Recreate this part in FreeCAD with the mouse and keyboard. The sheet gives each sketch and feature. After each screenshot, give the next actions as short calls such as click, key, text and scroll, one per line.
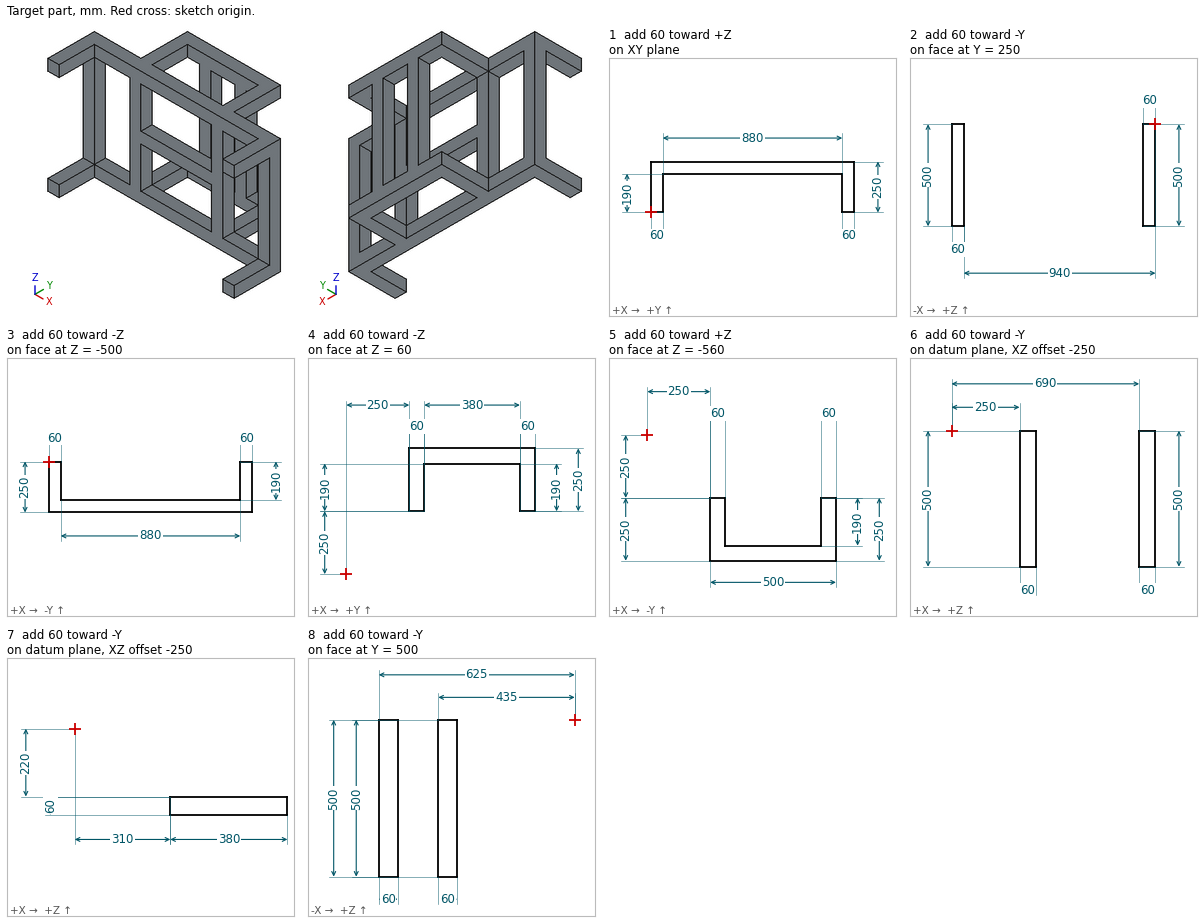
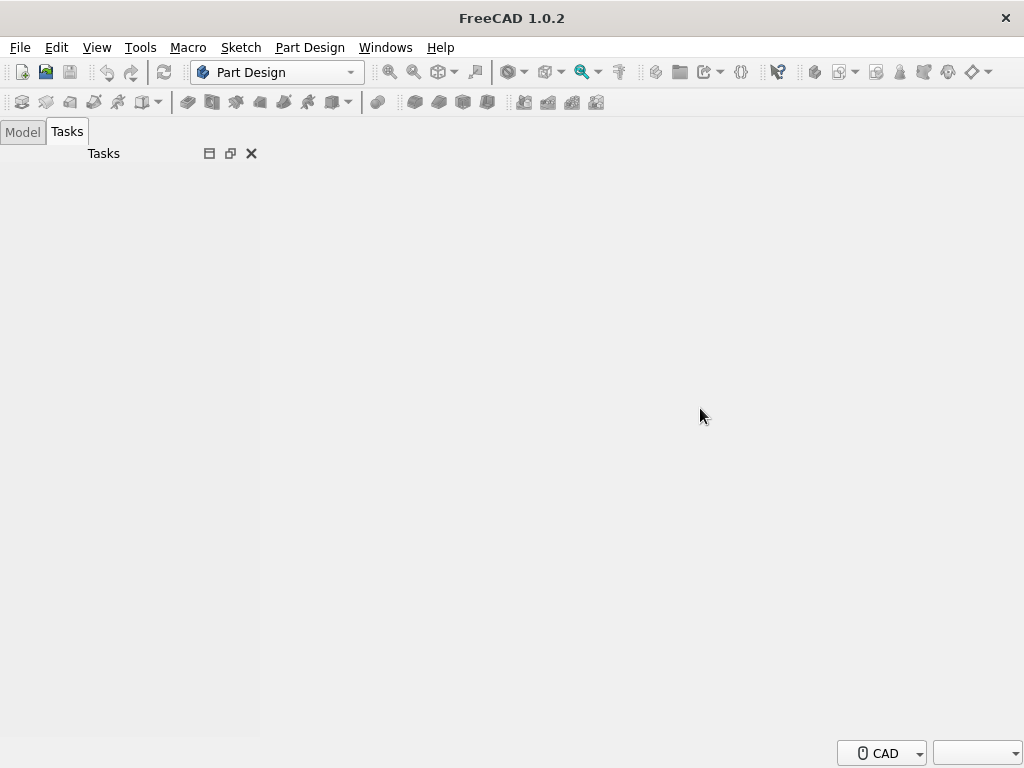
click(22, 72)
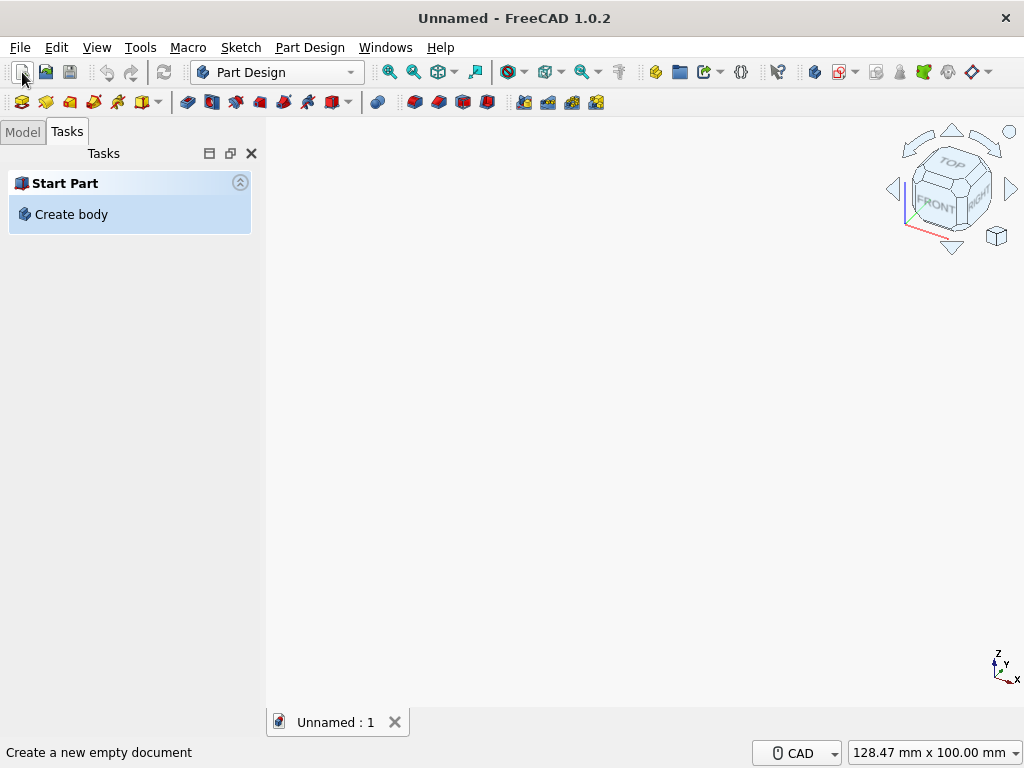
click(840, 72)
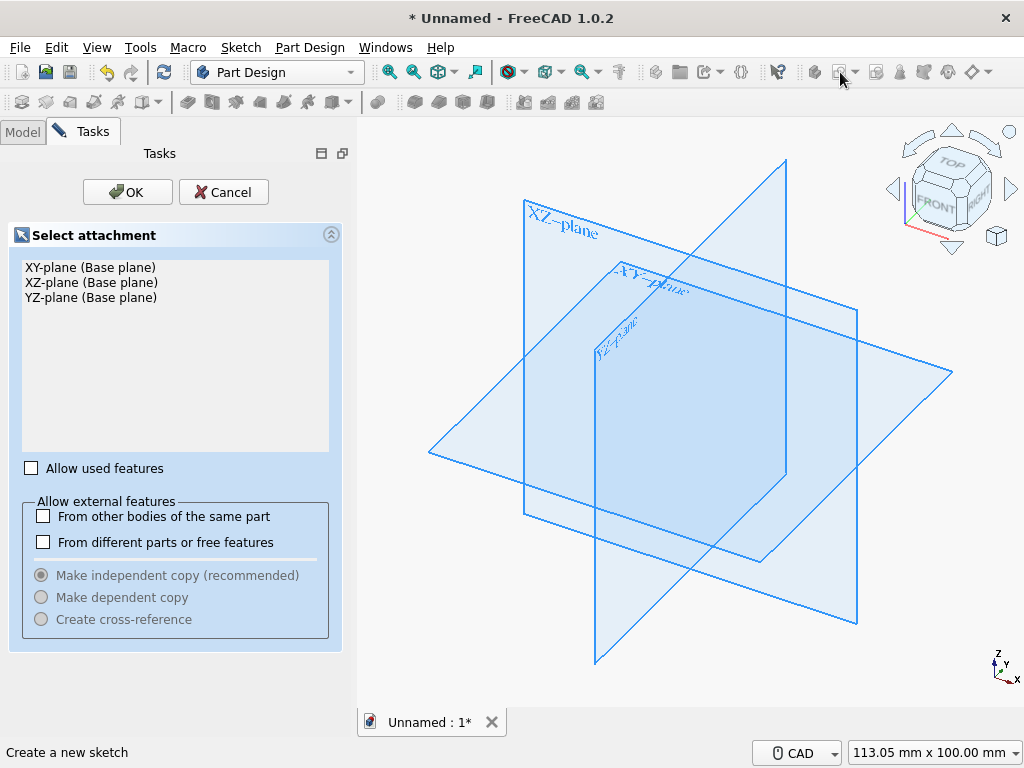
click(82, 268)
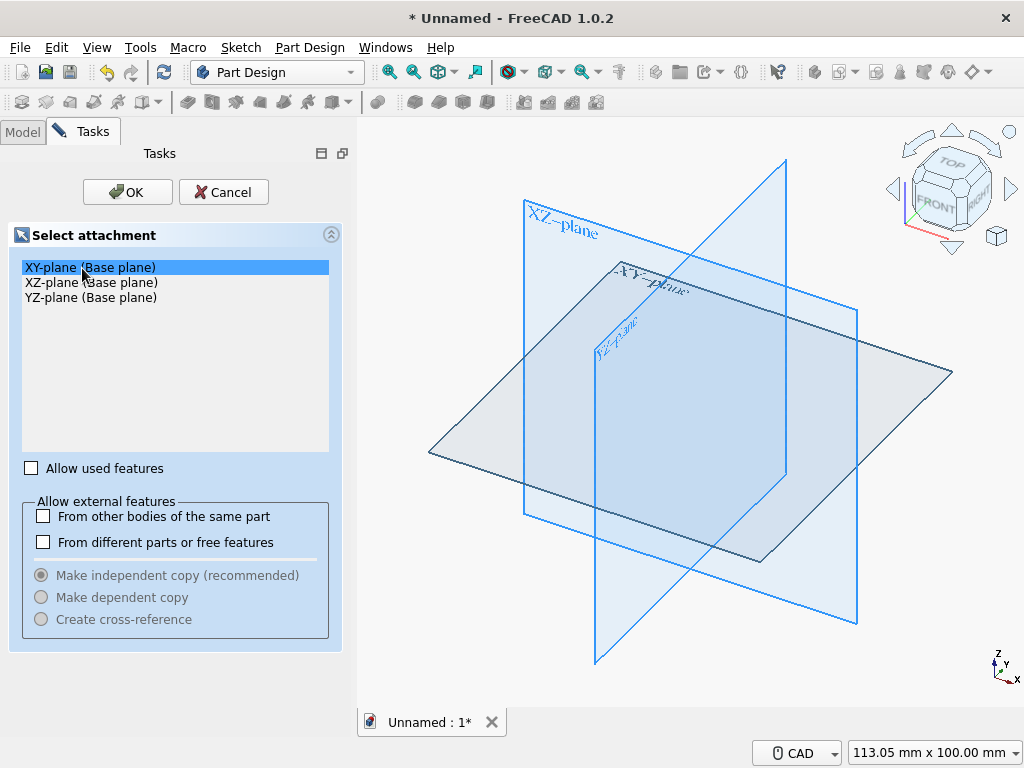
click(128, 192)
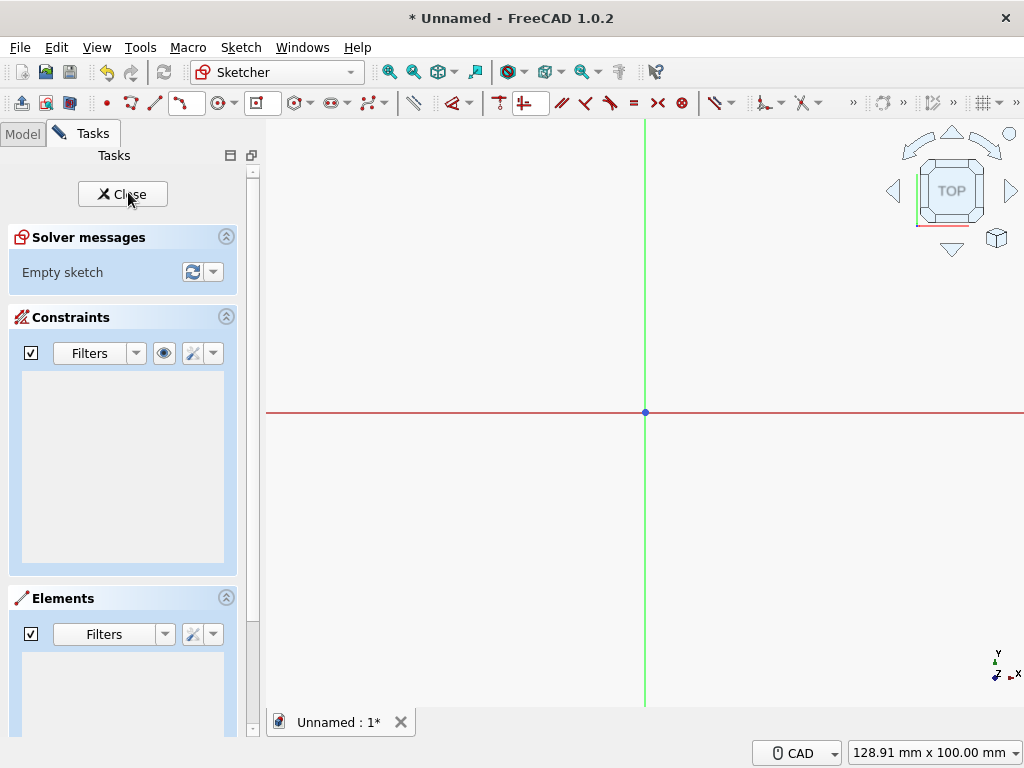
scroll(335, 472, down, 13)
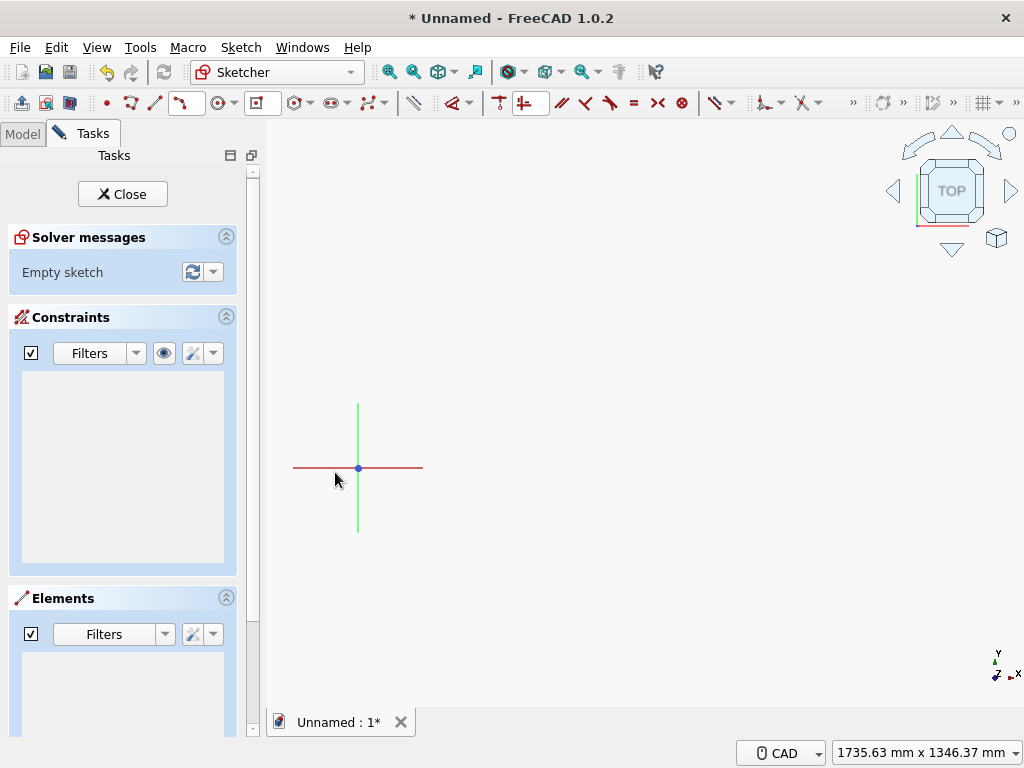
click(132, 104)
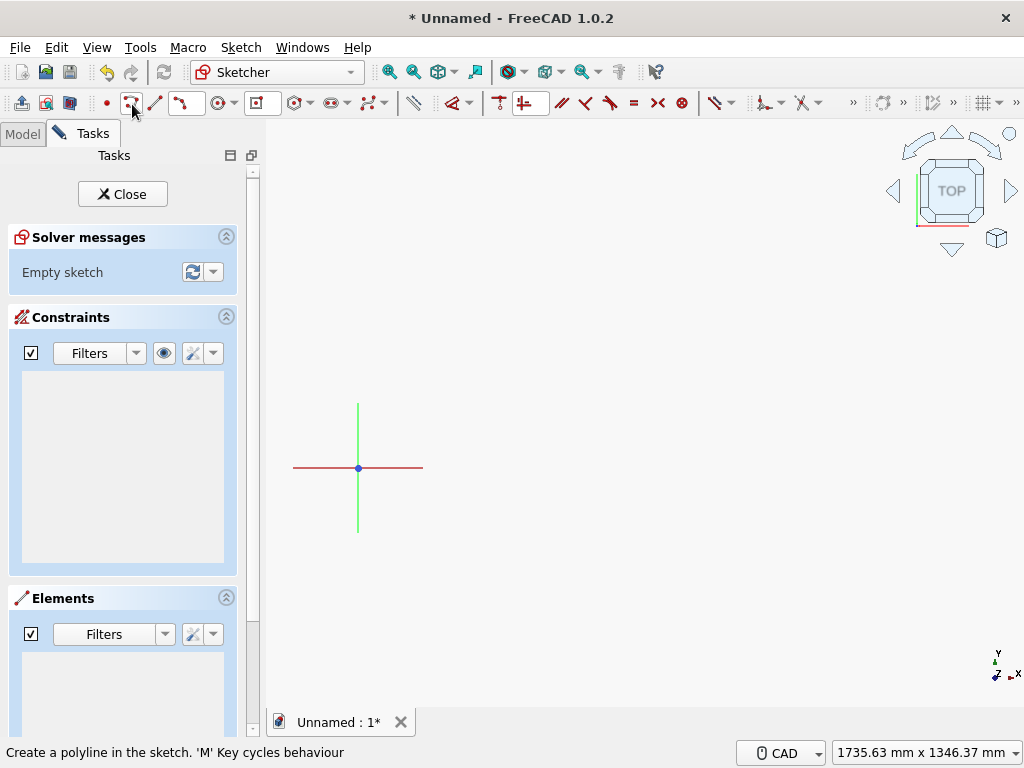
click(358, 468)
click(384, 459)
click(384, 385)
click(769, 385)
click(769, 468)
click(795, 459)
click(795, 359)
click(367, 359)
click(358, 468)
key(Escape)
key(Escape)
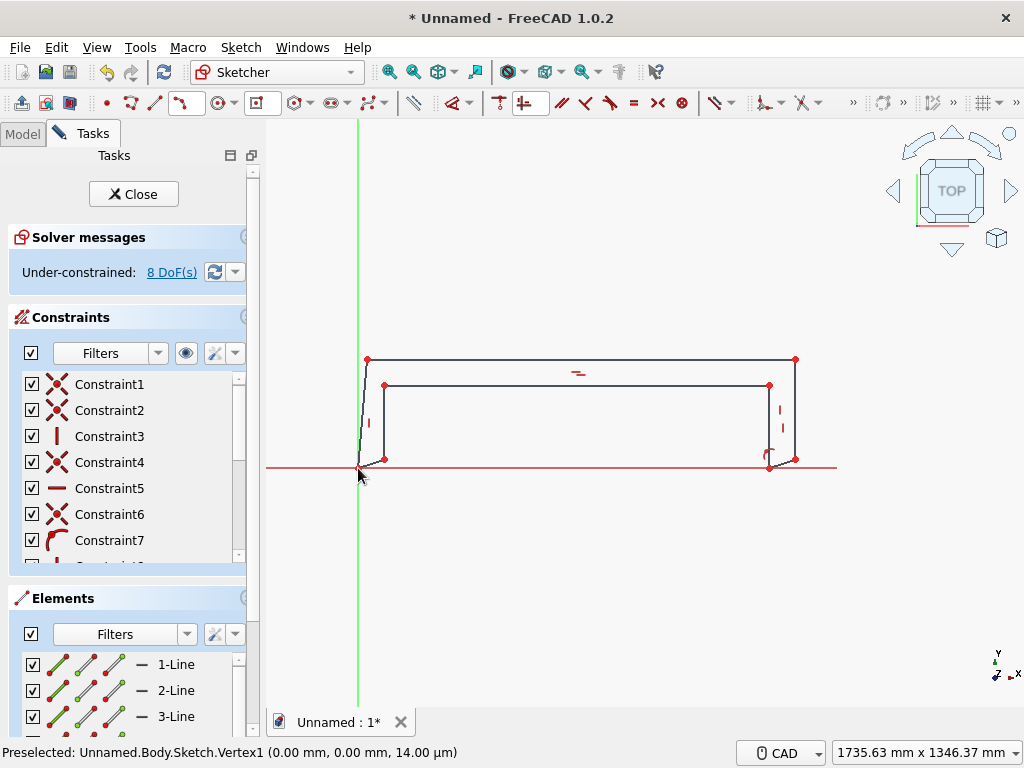
scroll(368, 465, up, 2)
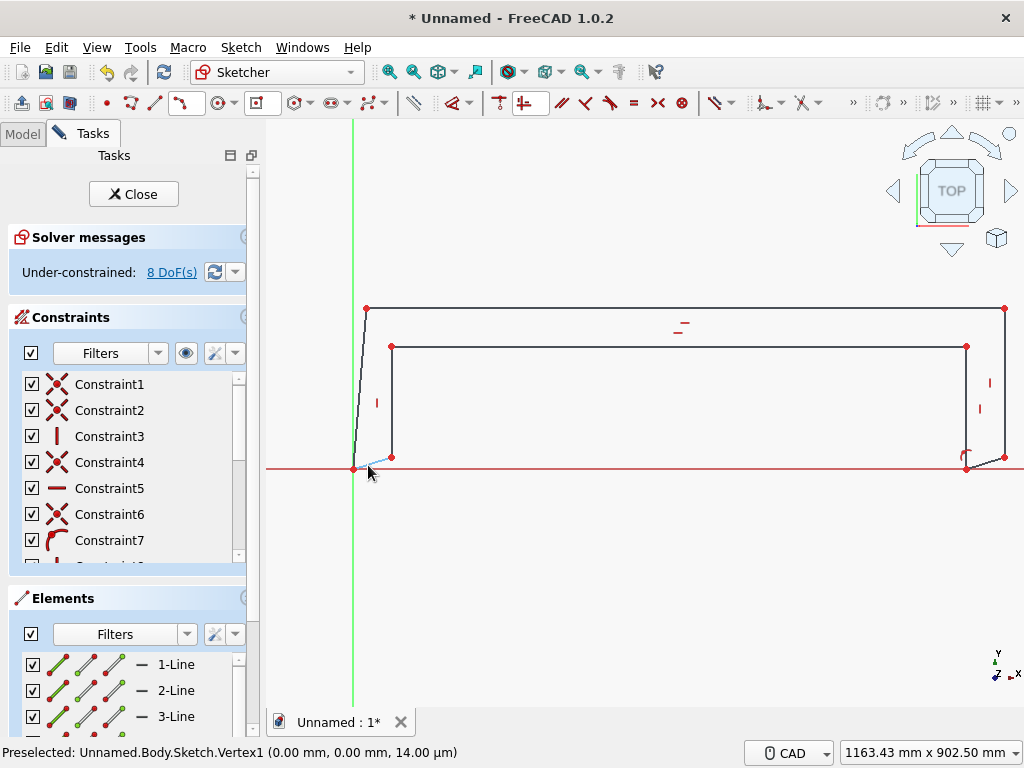
click(369, 465)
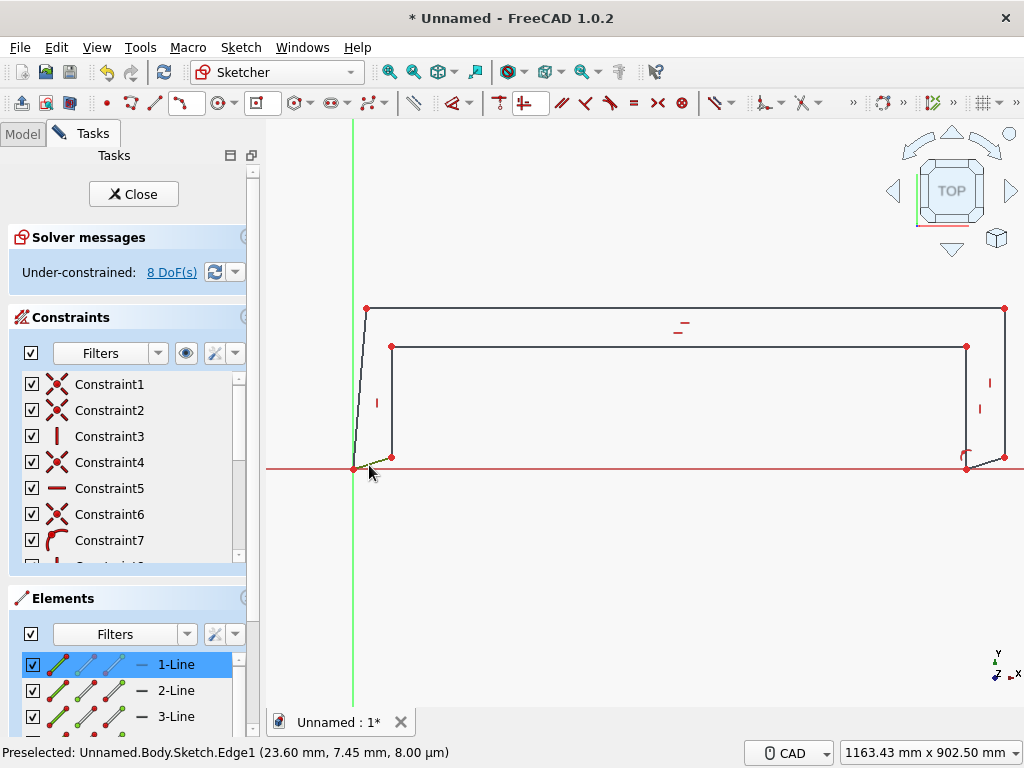
key(h)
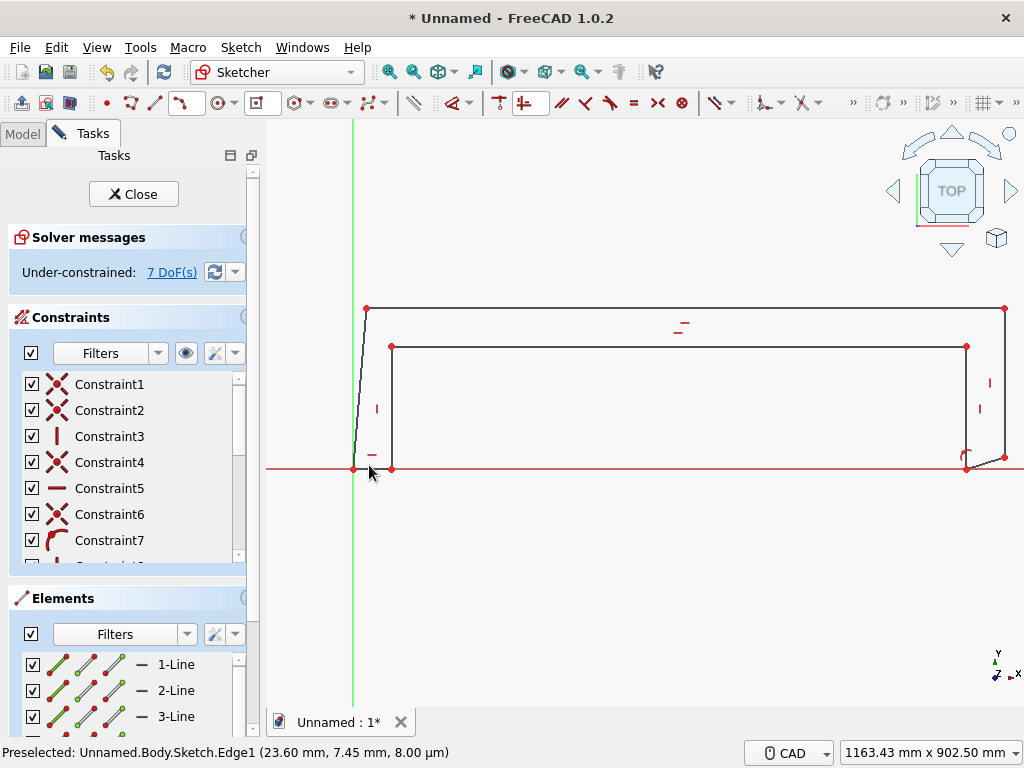
scroll(368, 464, down, 2)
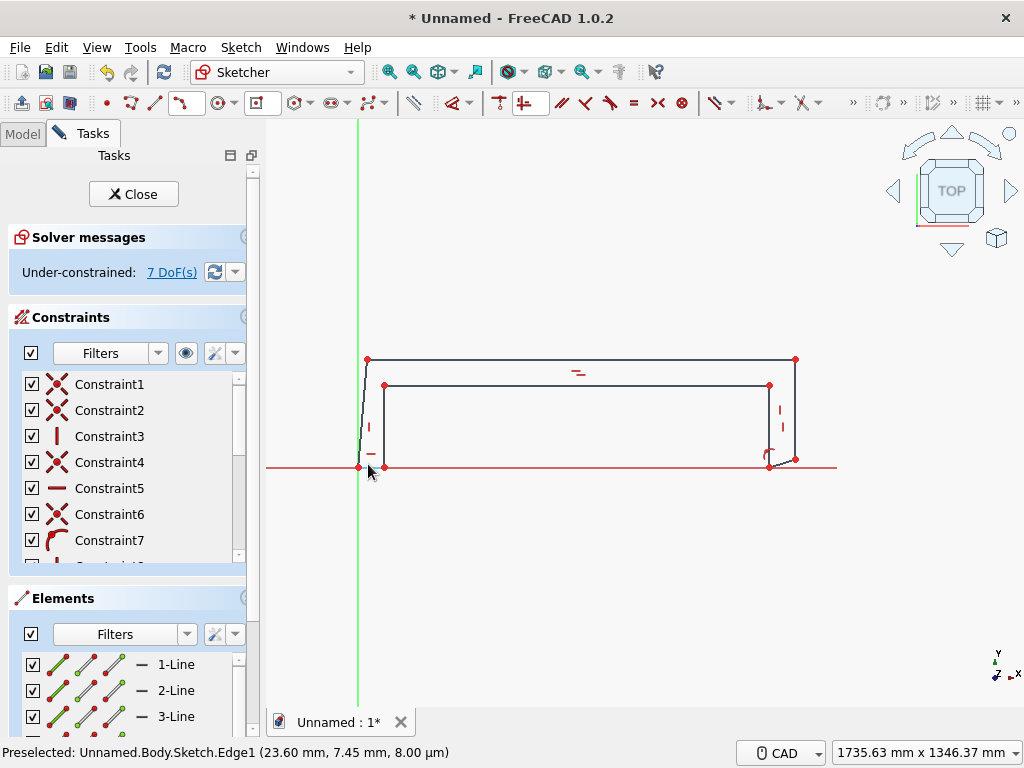
scroll(777, 465, up, 3)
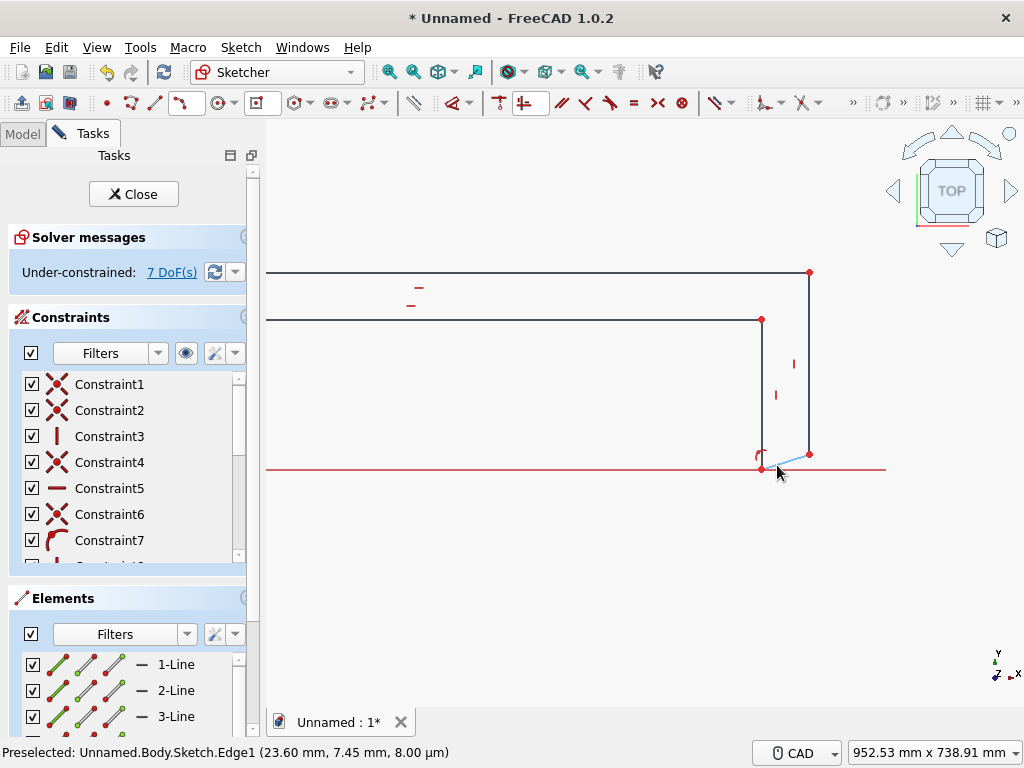
click(776, 465)